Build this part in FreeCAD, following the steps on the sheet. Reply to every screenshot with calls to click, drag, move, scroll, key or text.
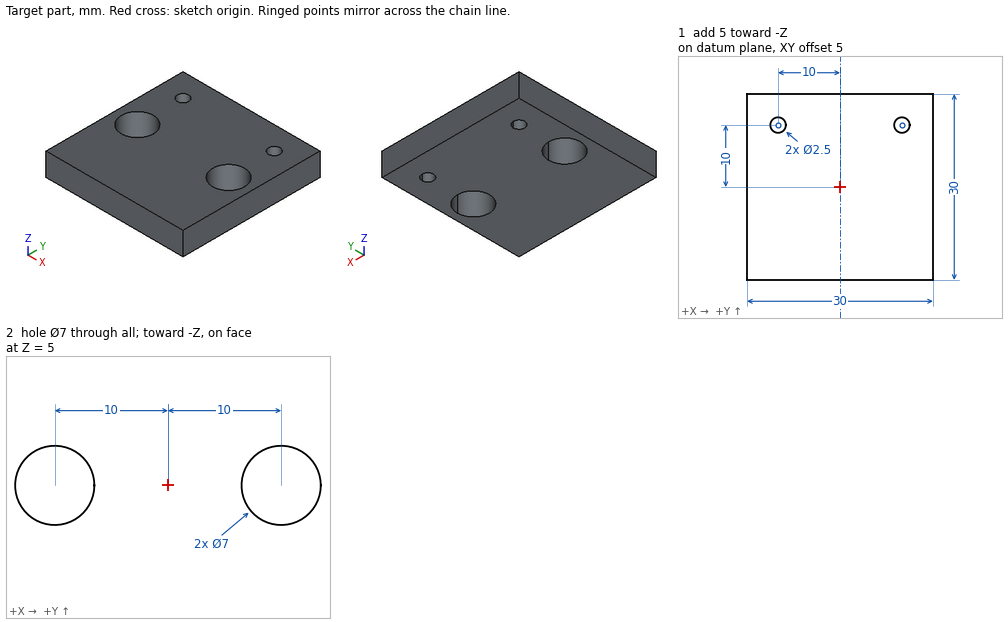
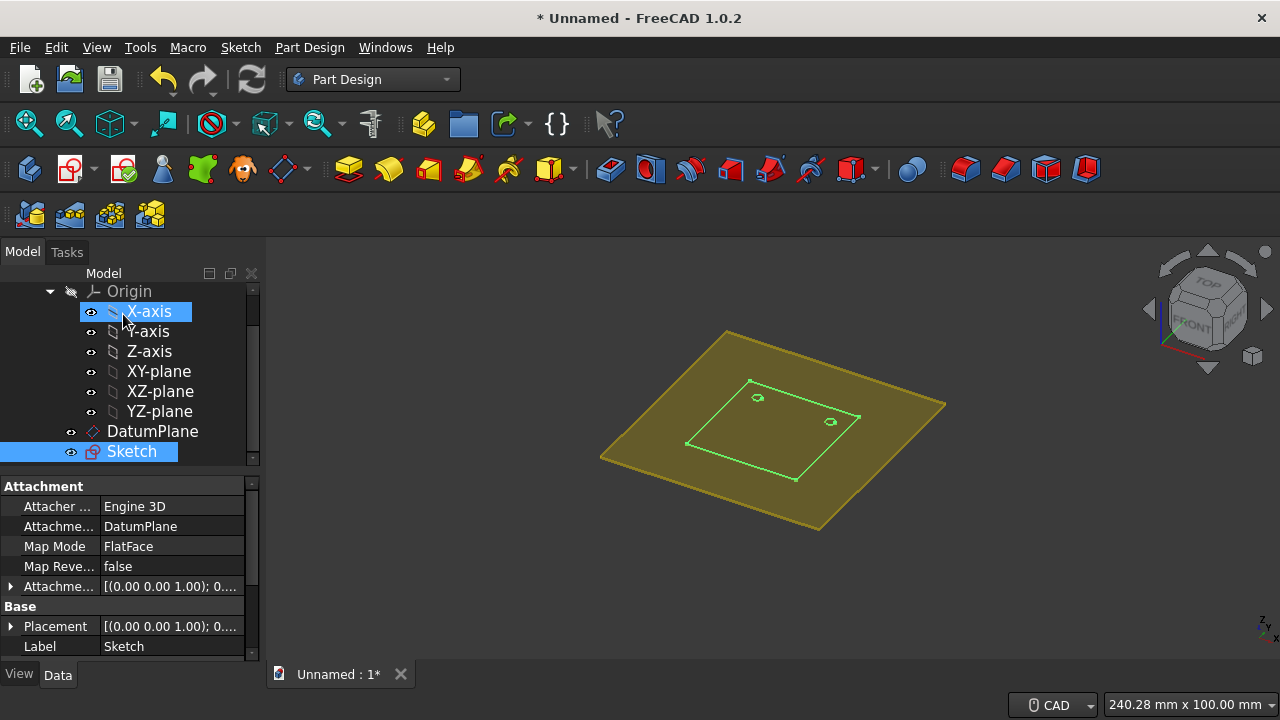
click(350, 170)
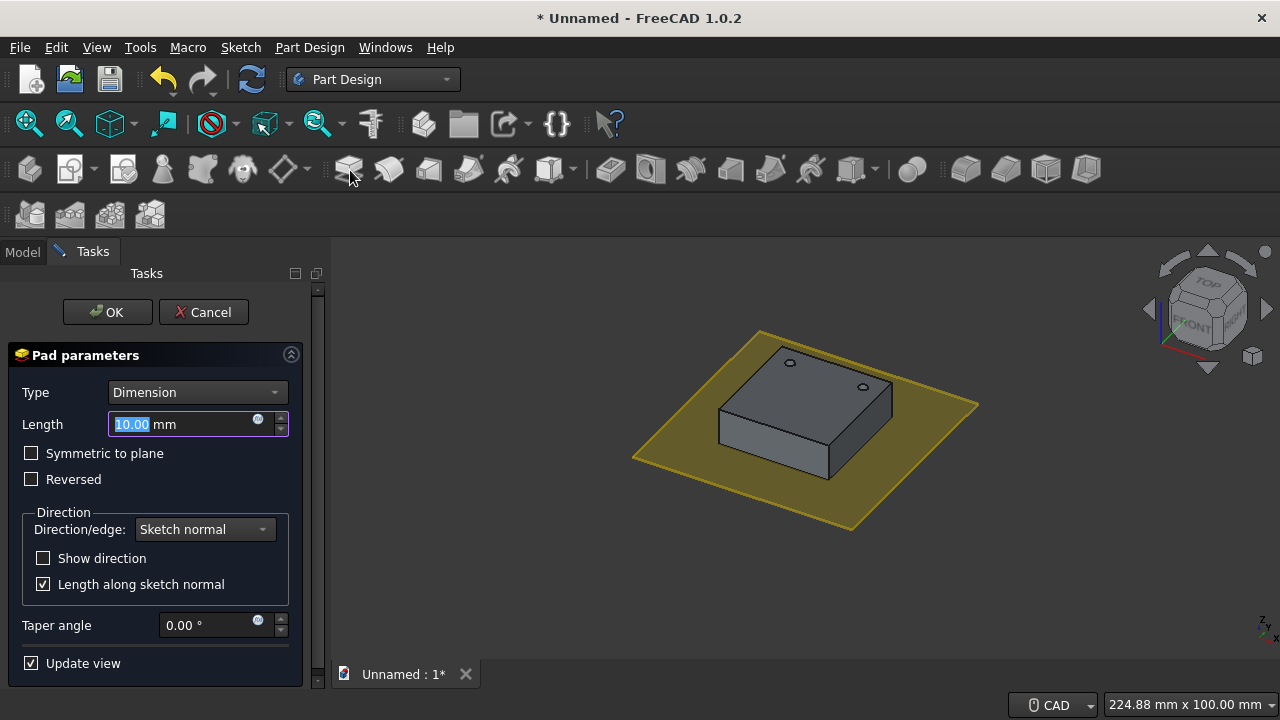
text(5)
key(Tab)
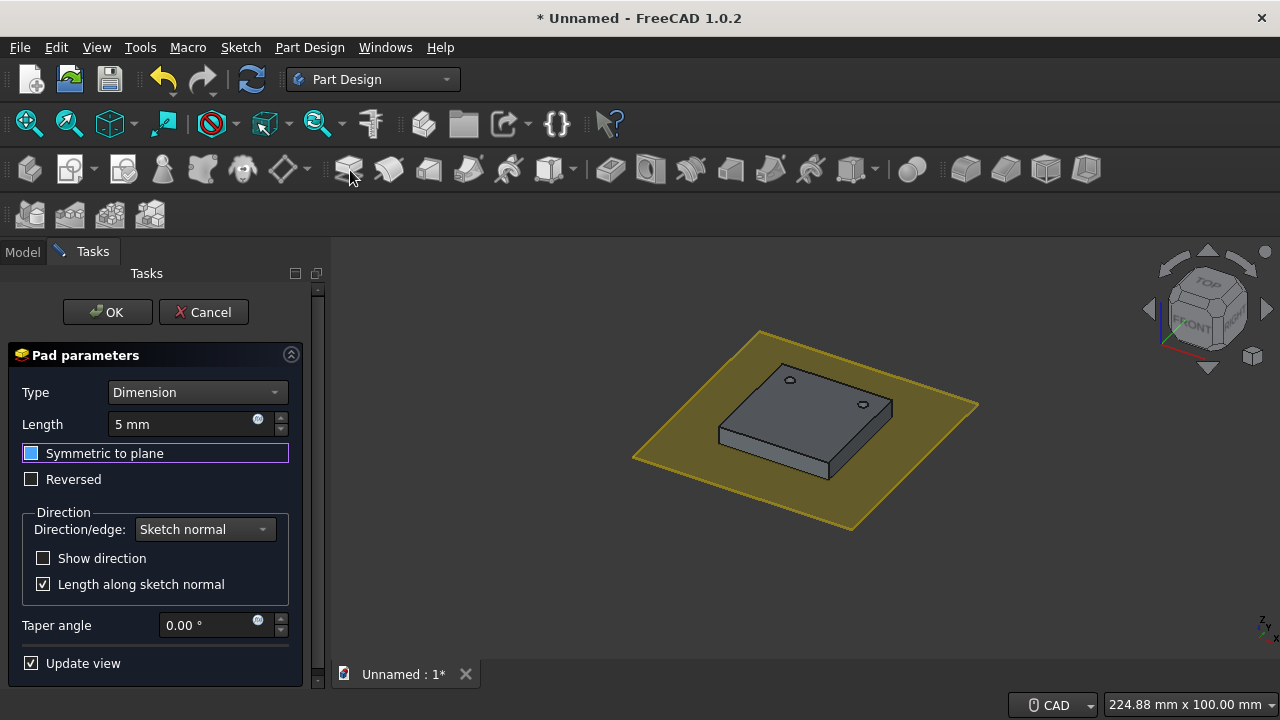
click(30, 479)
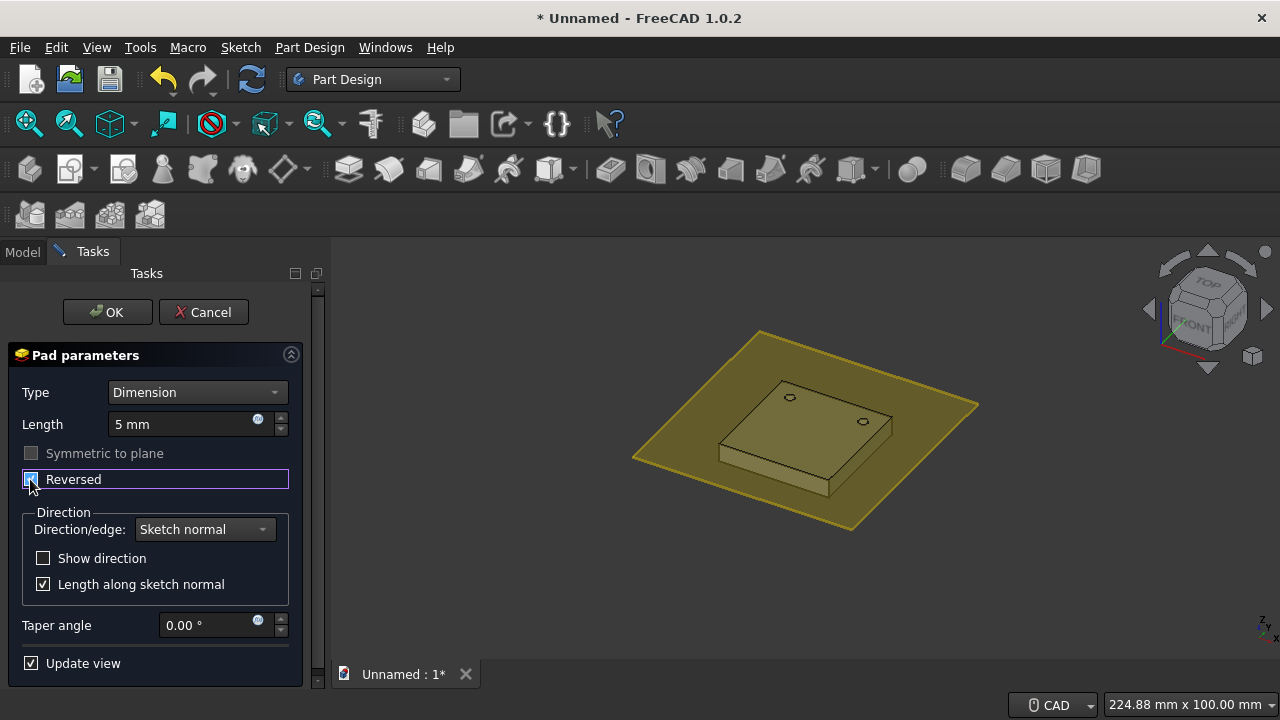
click(108, 312)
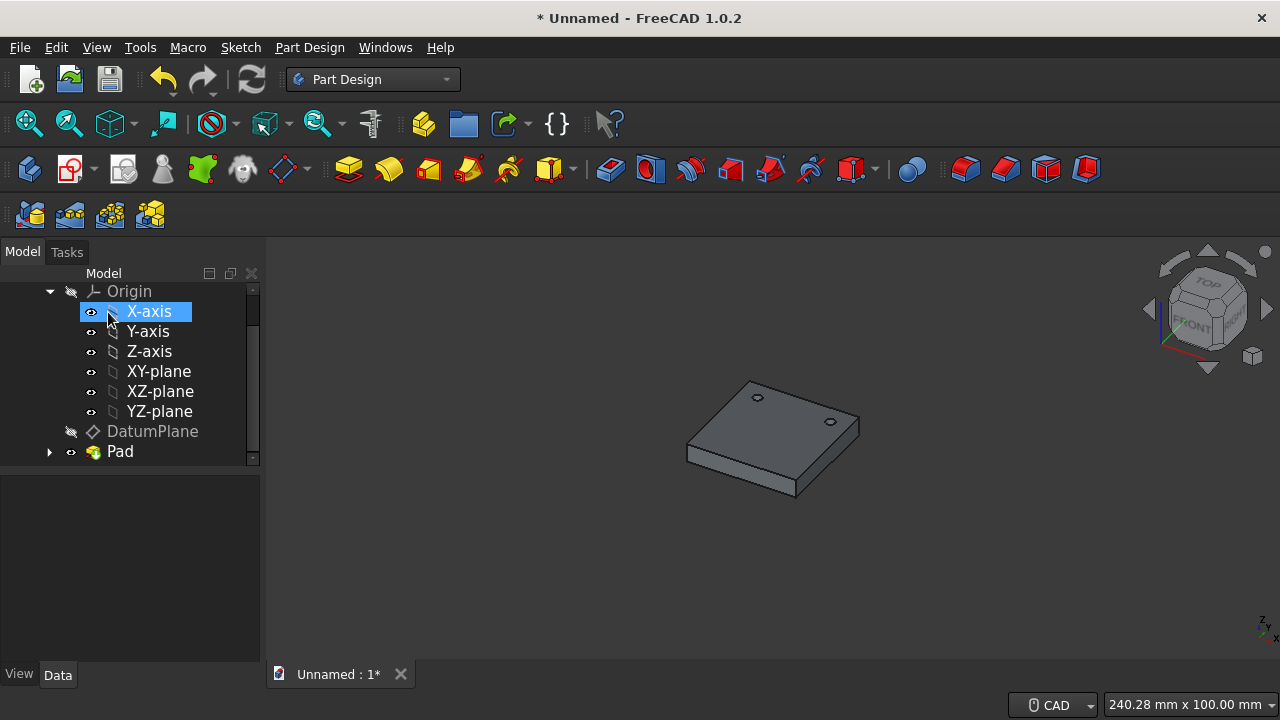
click(30, 124)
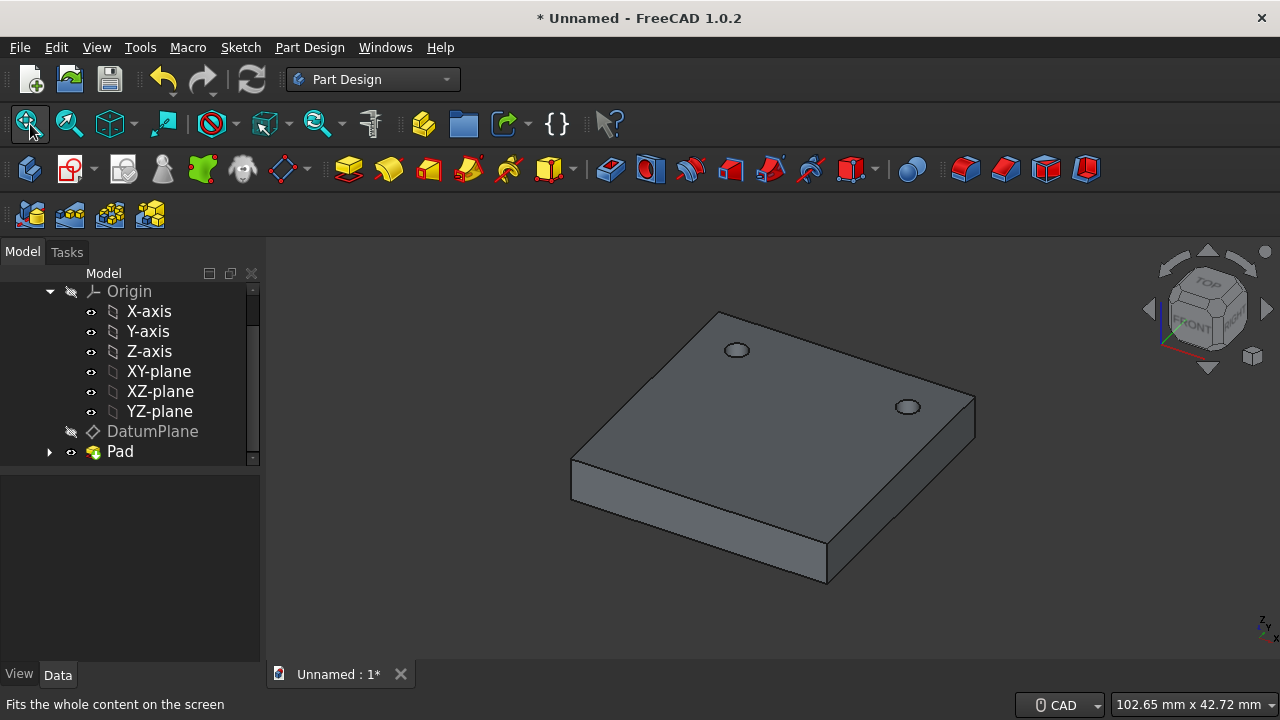
click(773, 427)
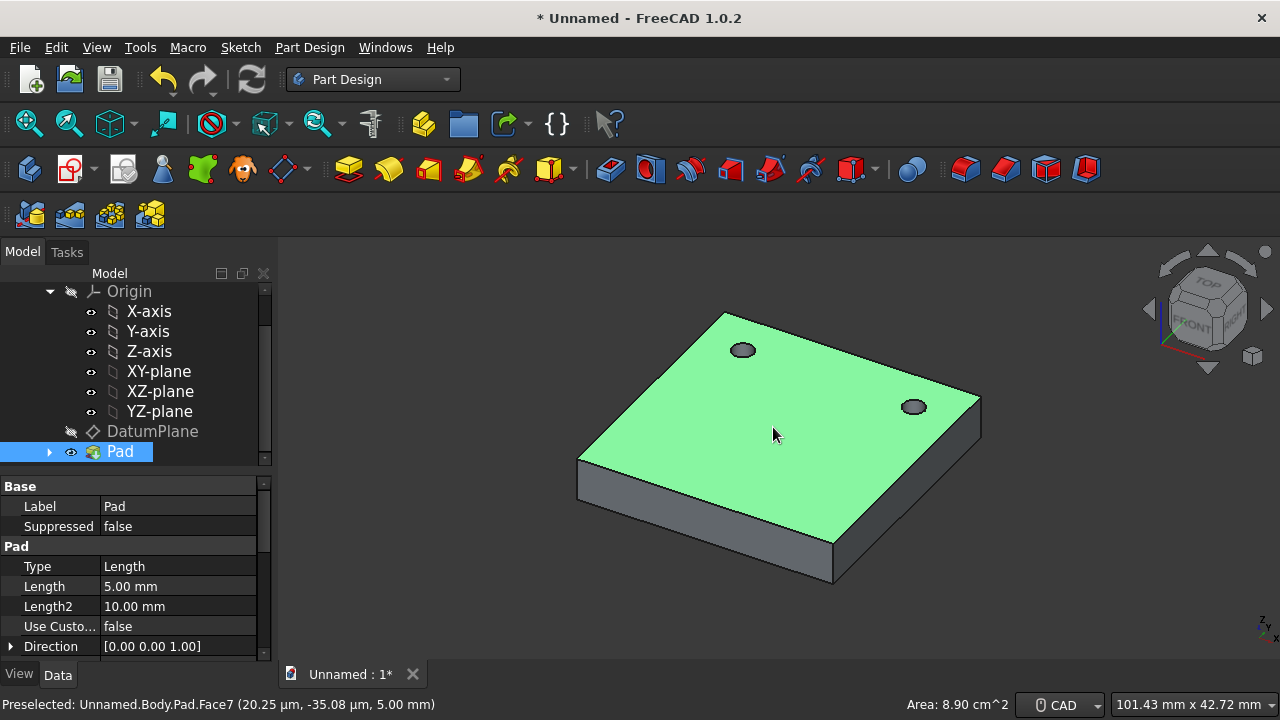
click(70, 170)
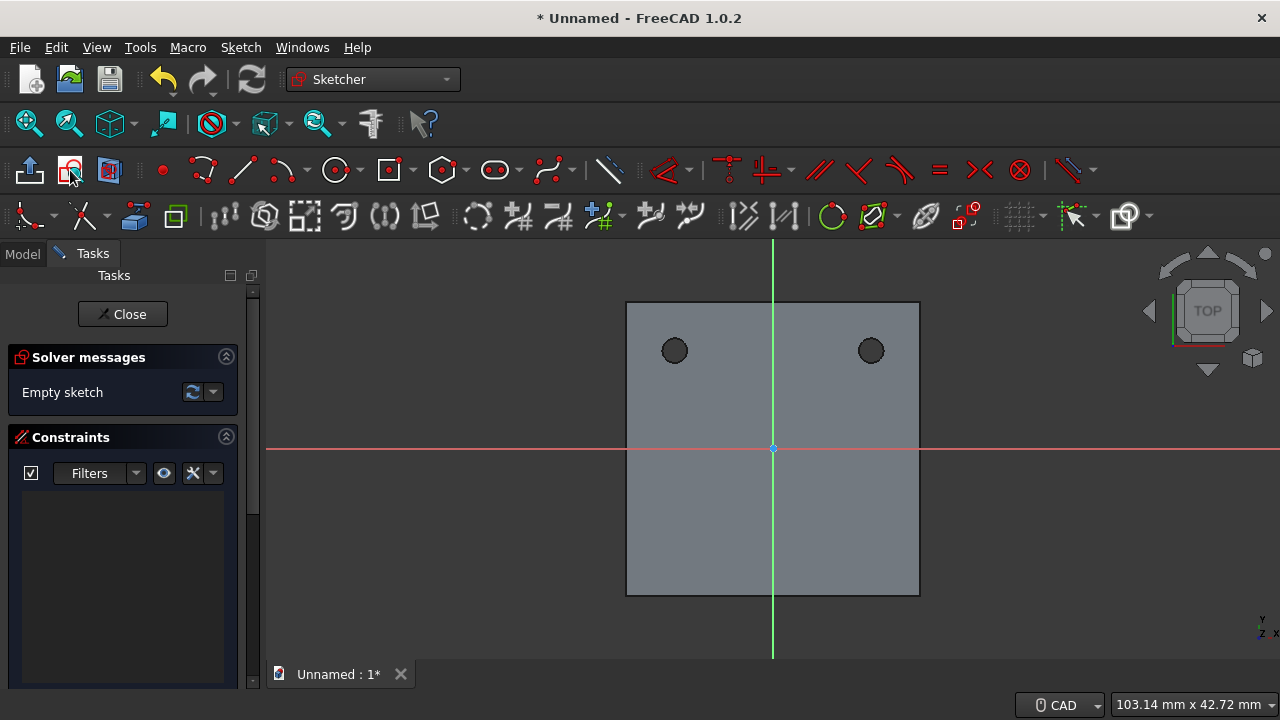
scroll(829, 449, up, 4)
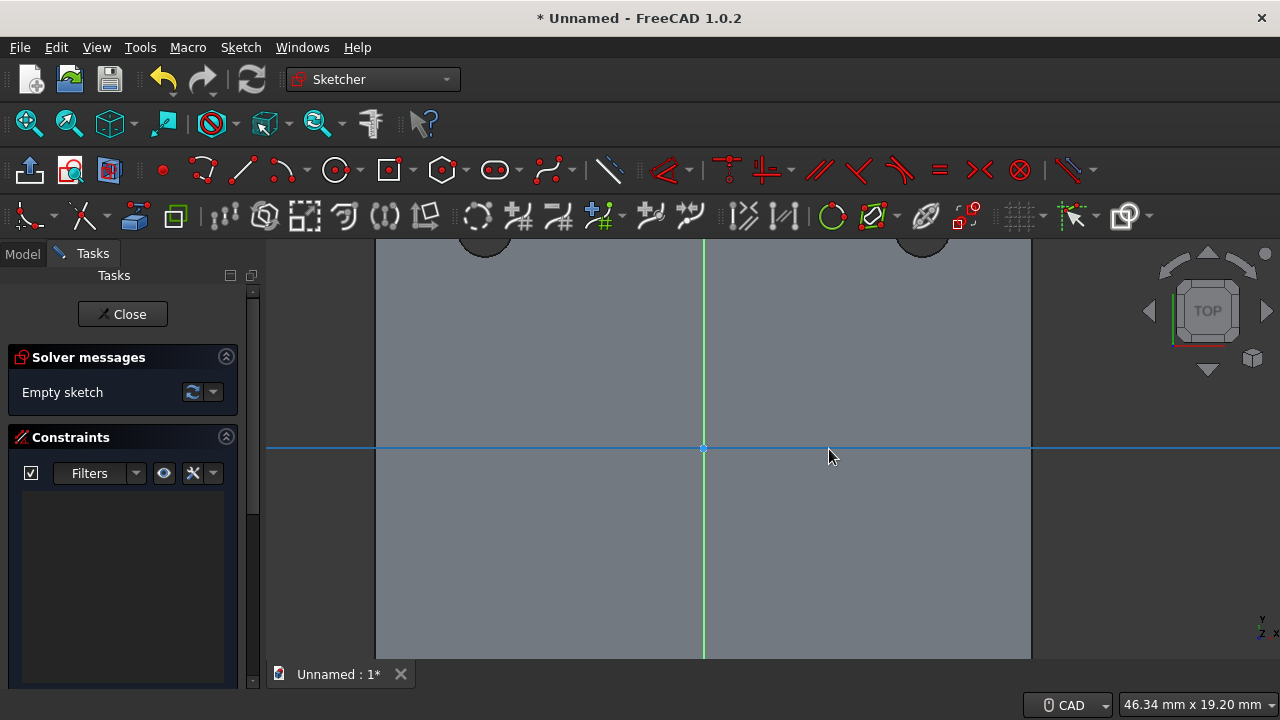
click(336, 170)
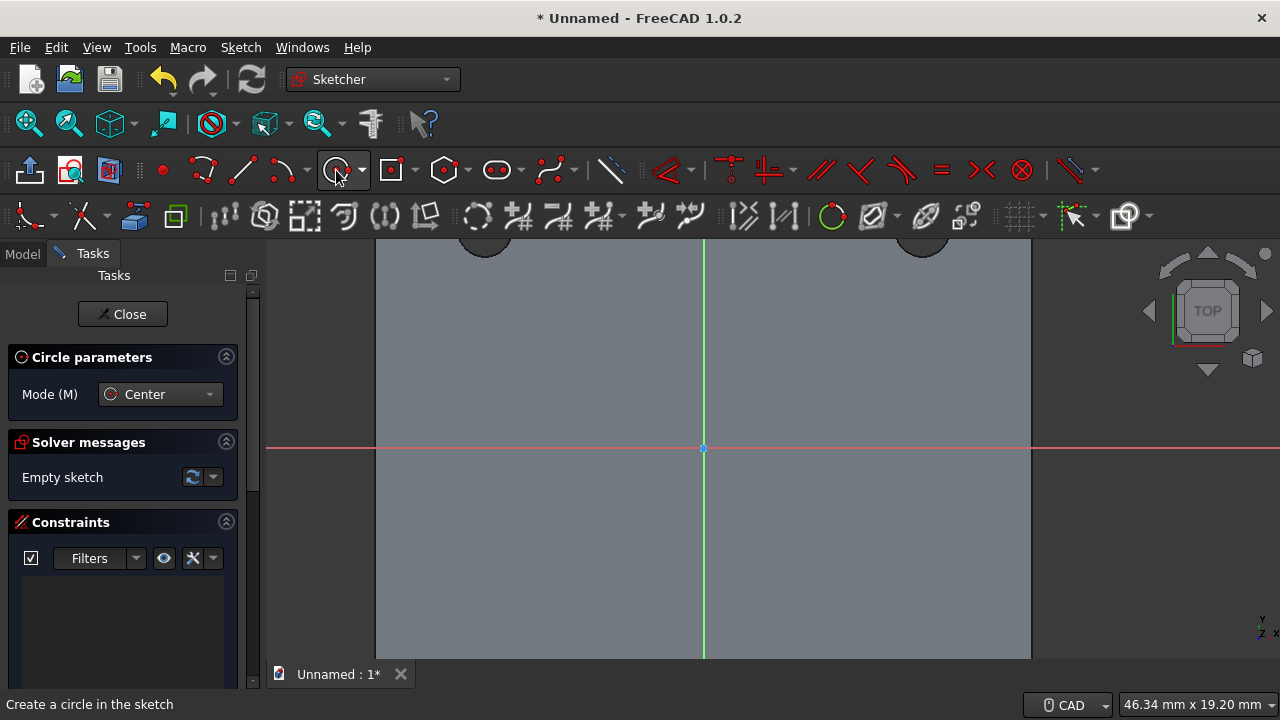
click(922, 448)
move(977, 394)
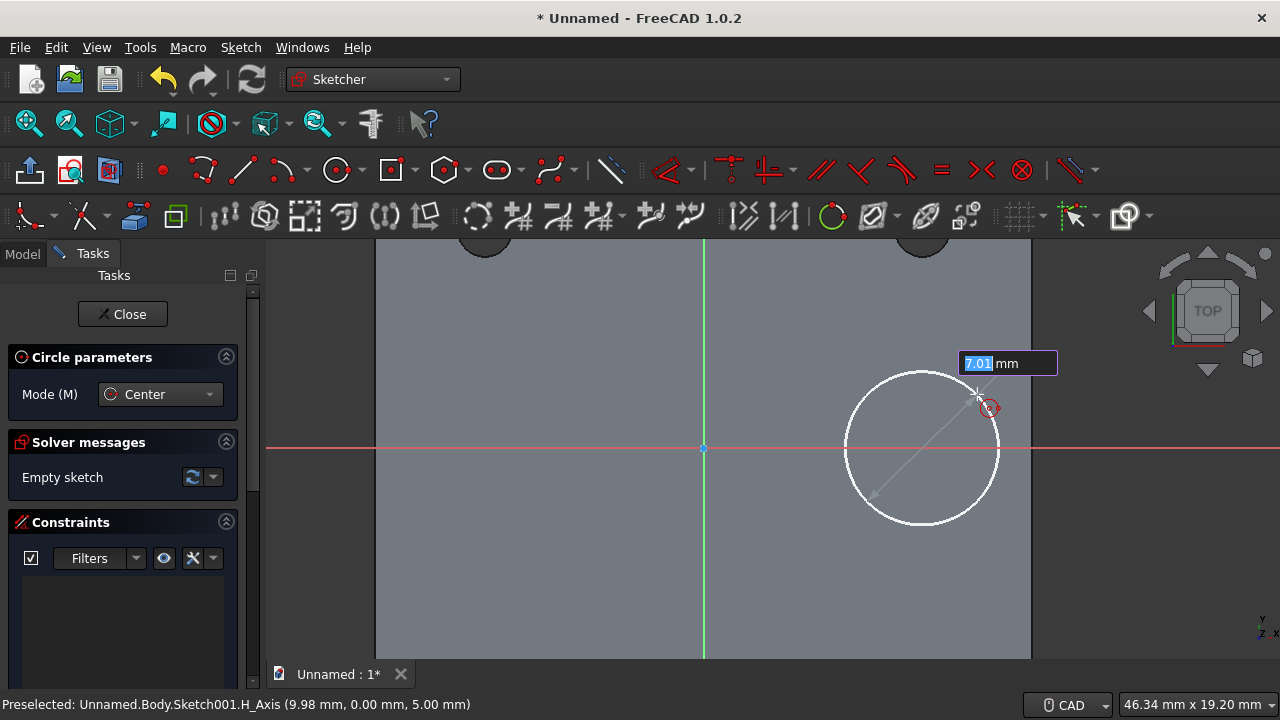
text(7)
key(Return)